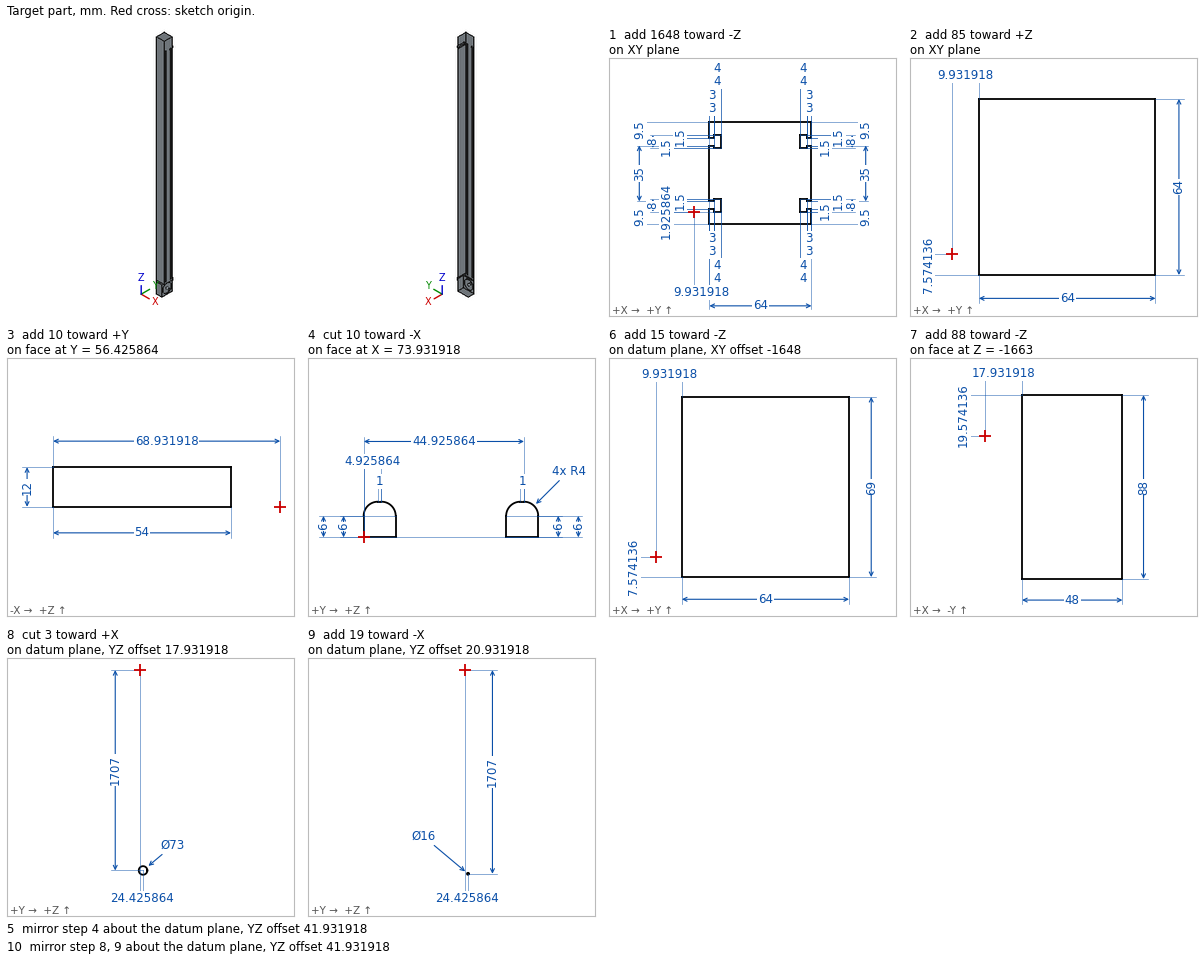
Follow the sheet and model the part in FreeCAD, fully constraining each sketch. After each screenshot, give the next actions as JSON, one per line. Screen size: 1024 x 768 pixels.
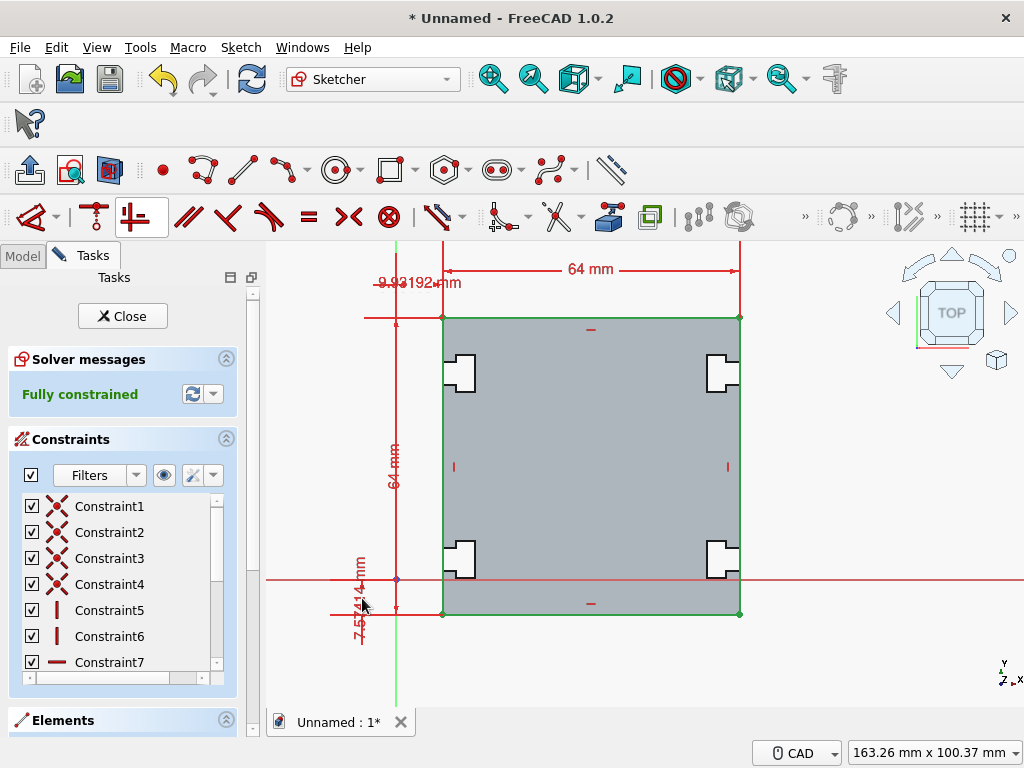
{"action": "left_click", "coordinate": [123, 316]}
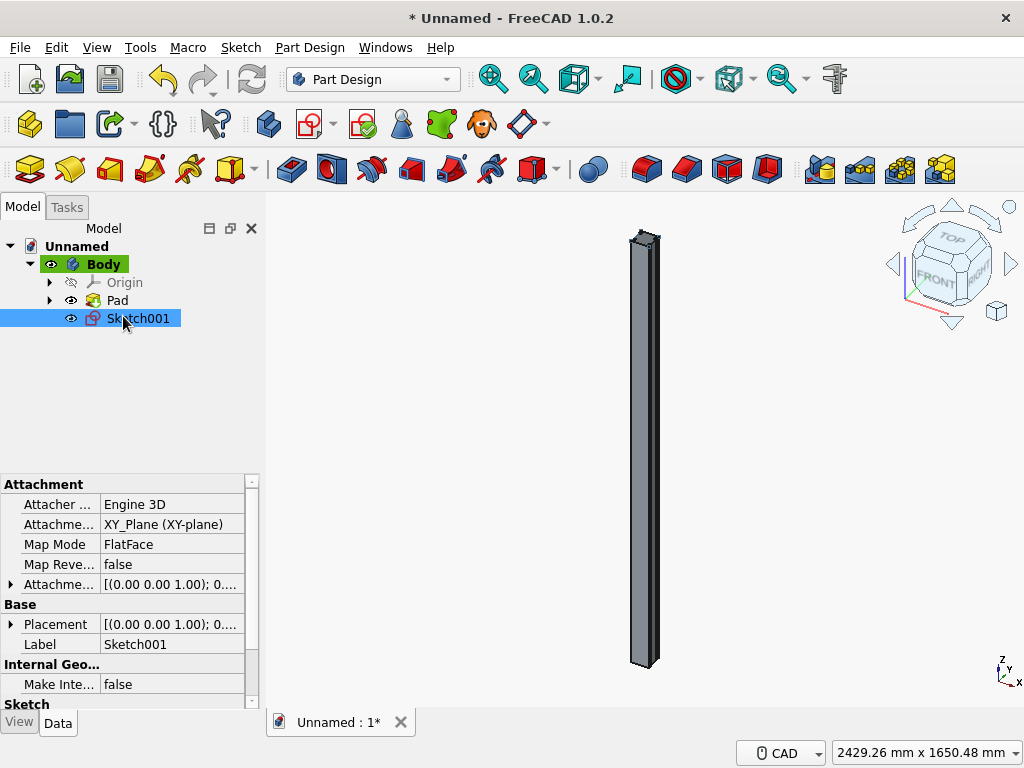
{"action": "left_click", "coordinate": [30, 170]}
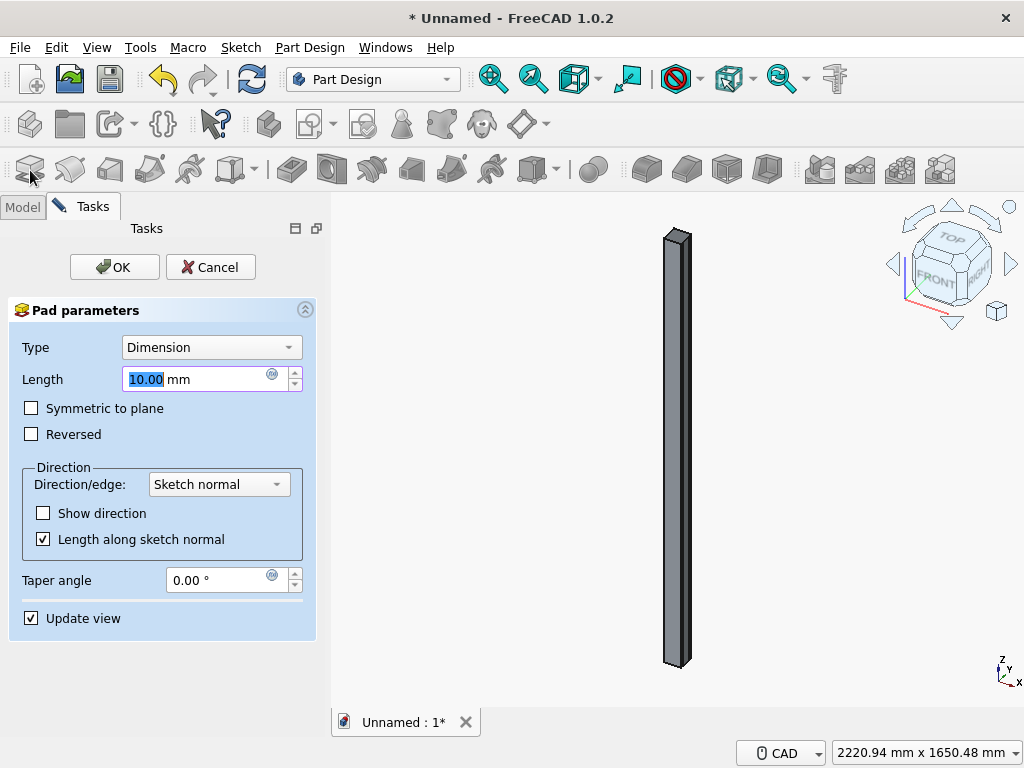
{"action": "type", "text": "85"}
{"action": "key", "text": "Tab"}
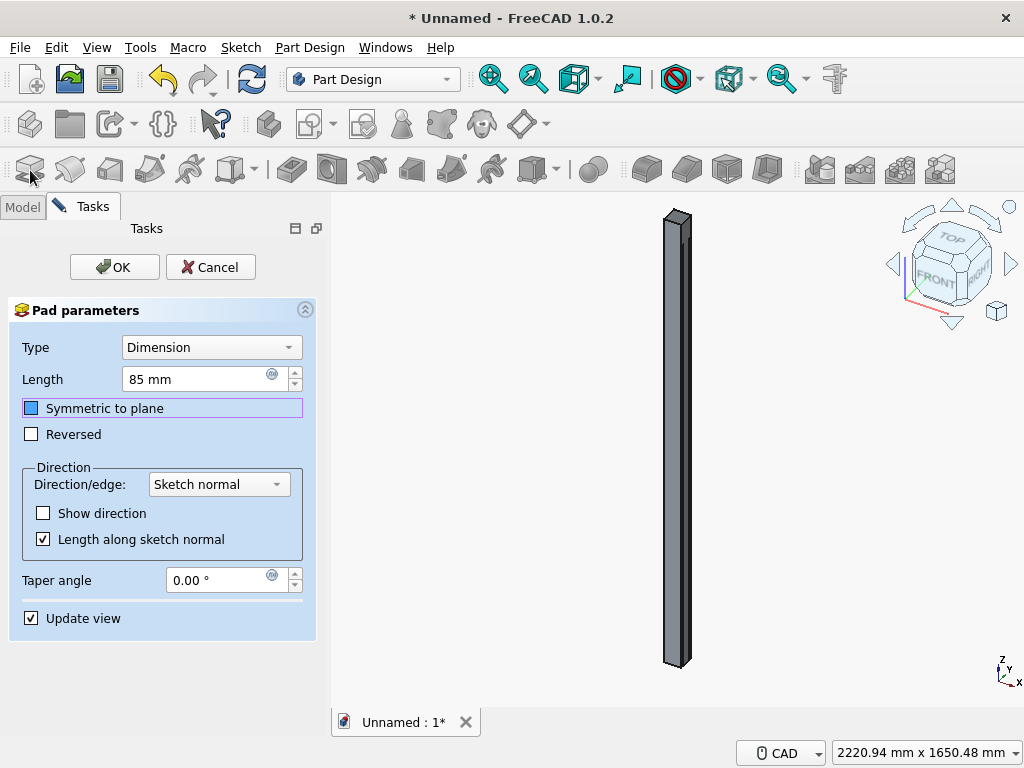
{"action": "left_click", "coordinate": [115, 267]}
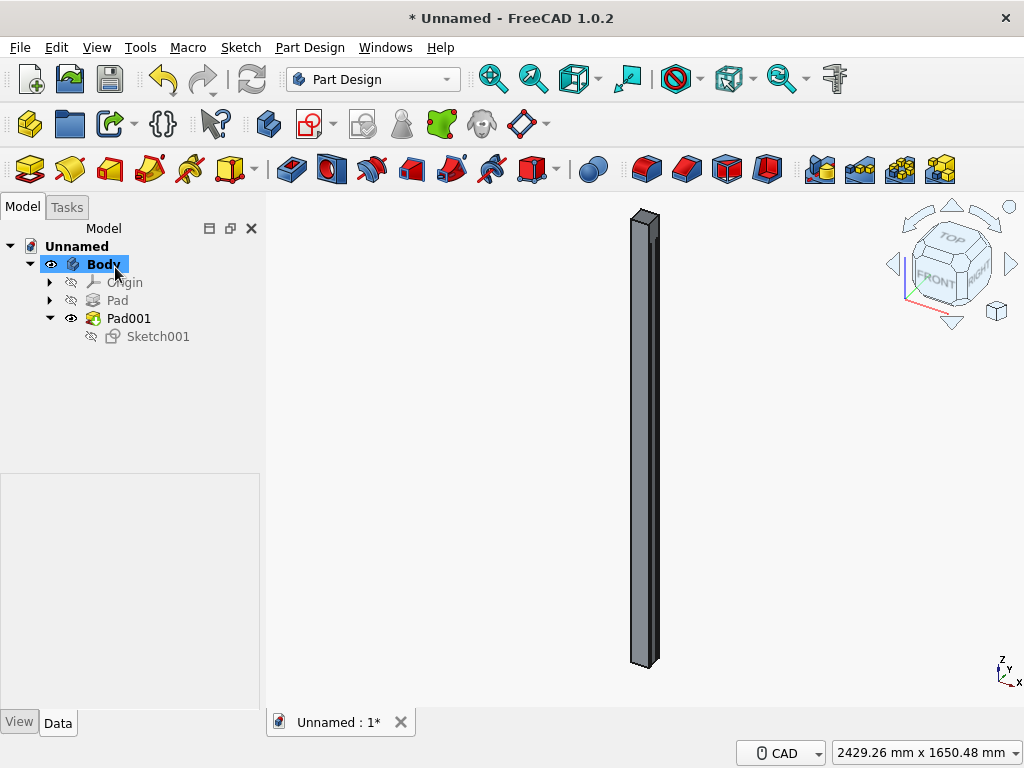
{"action": "key", "text": "4"}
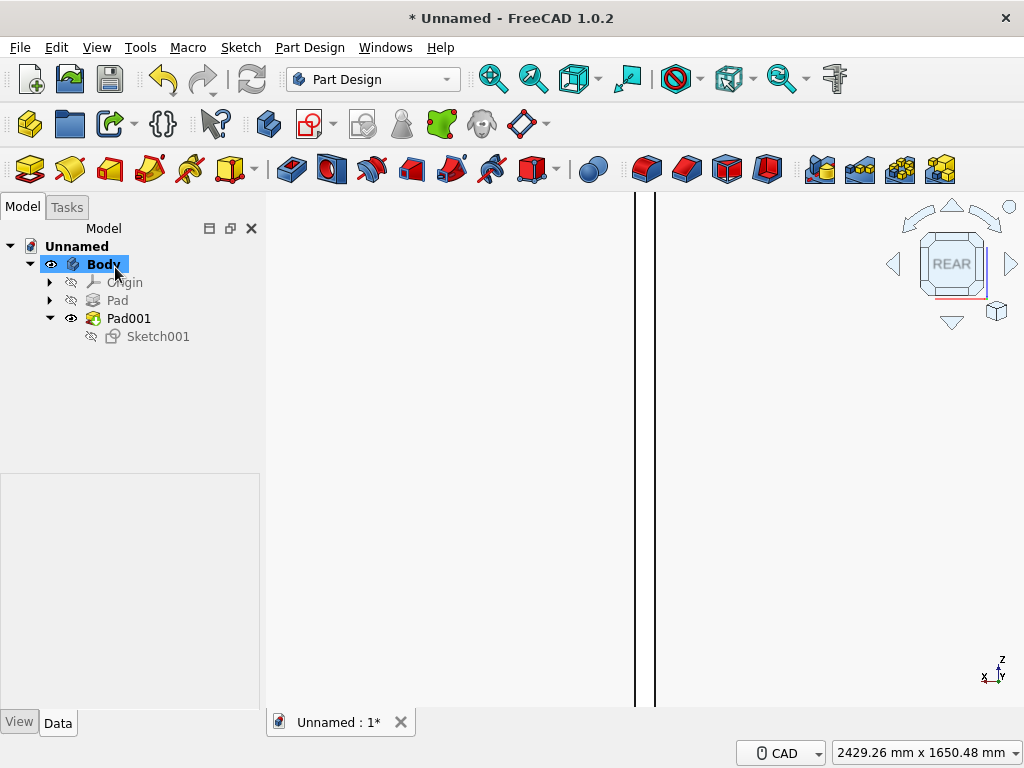
{"action": "left_click", "coordinate": [494, 80]}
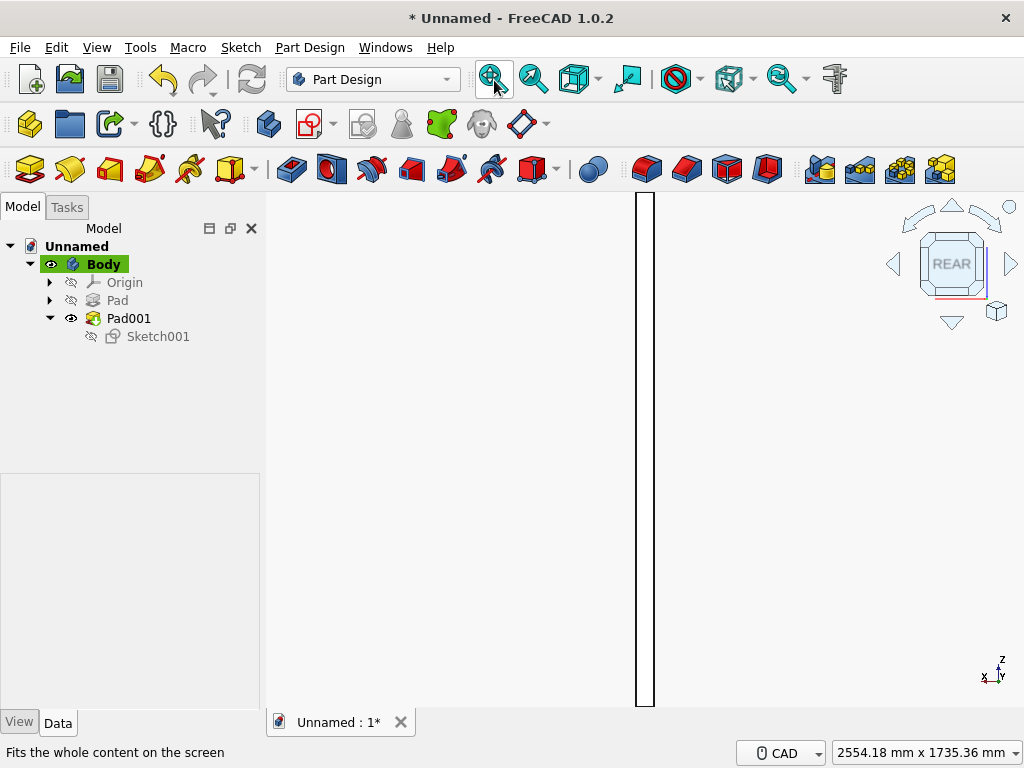
{"action": "left_click", "coordinate": [645, 228]}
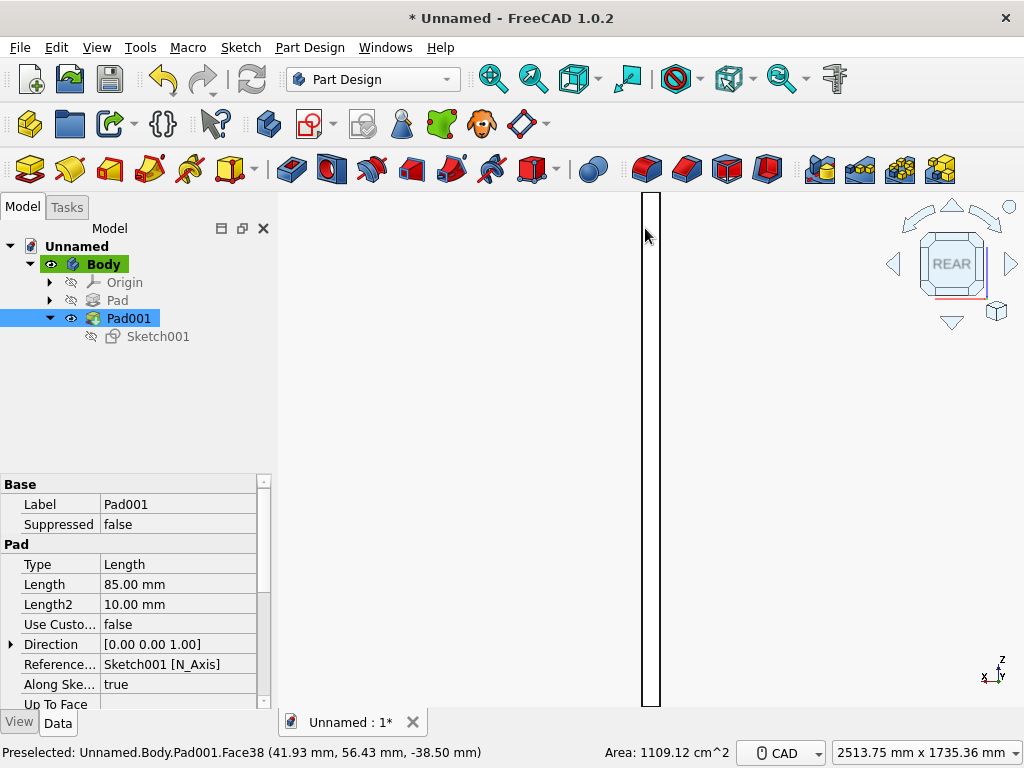
{"action": "left_click", "coordinate": [310, 124]}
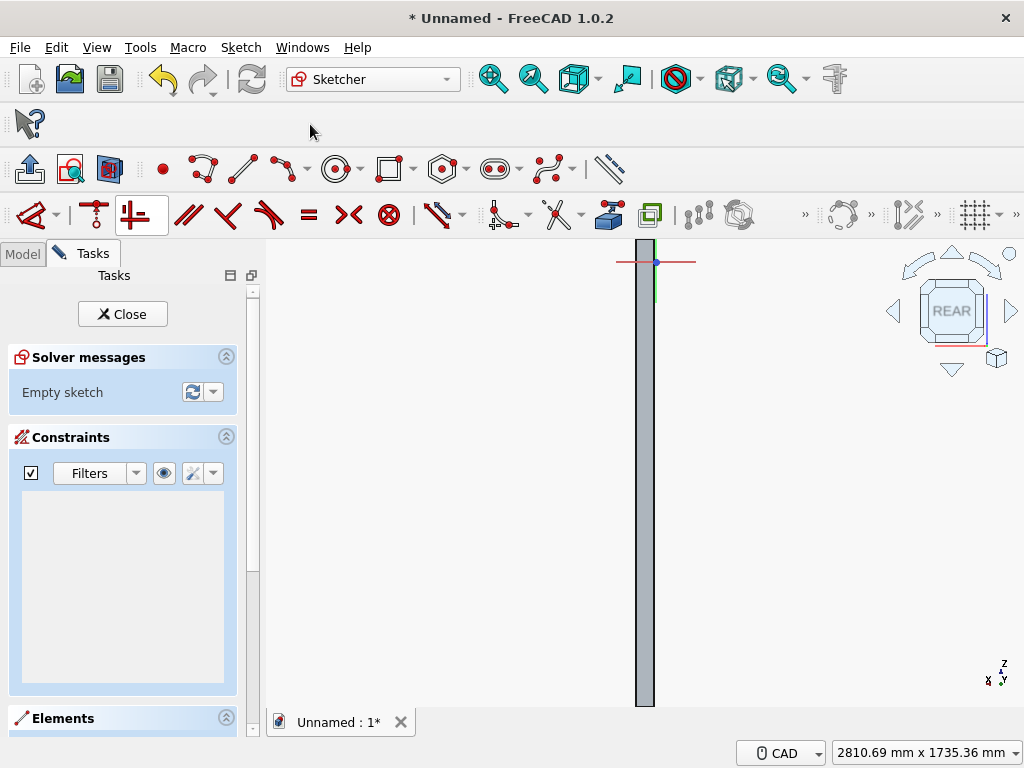
{"action": "scroll", "coordinate": [576, 473], "scroll_direction": "down", "scroll_amount": 5}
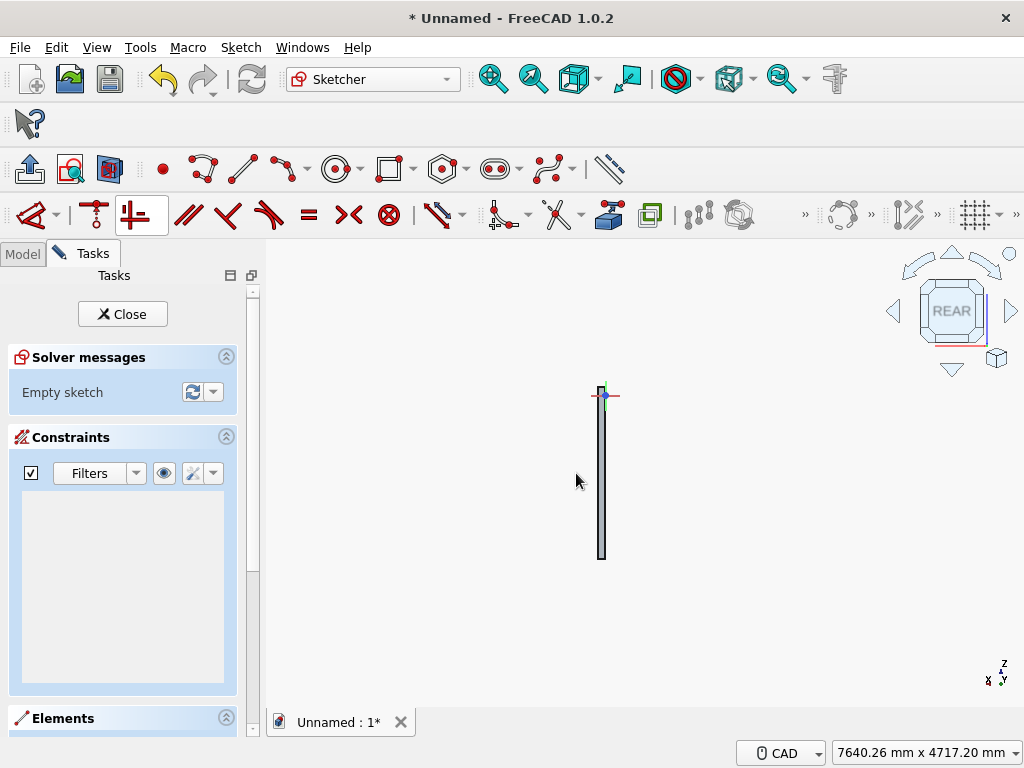
{"action": "scroll", "coordinate": [604, 391], "scroll_direction": "up", "scroll_amount": 15}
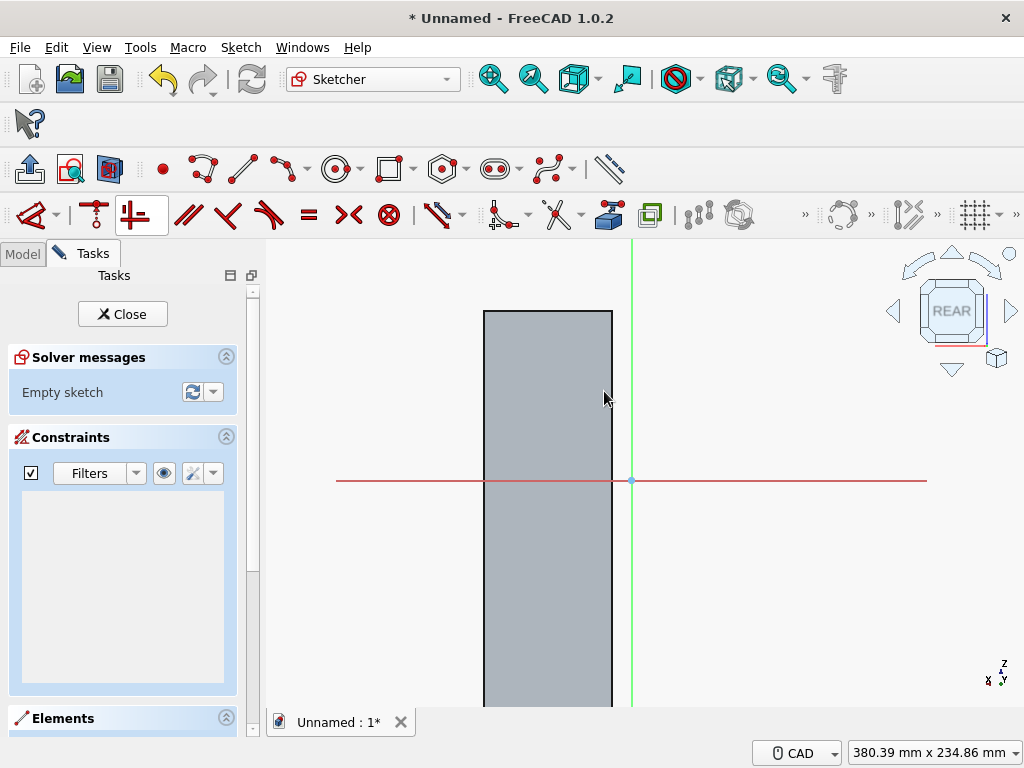
{"action": "scroll", "coordinate": [555, 467], "scroll_direction": "up", "scroll_amount": 5}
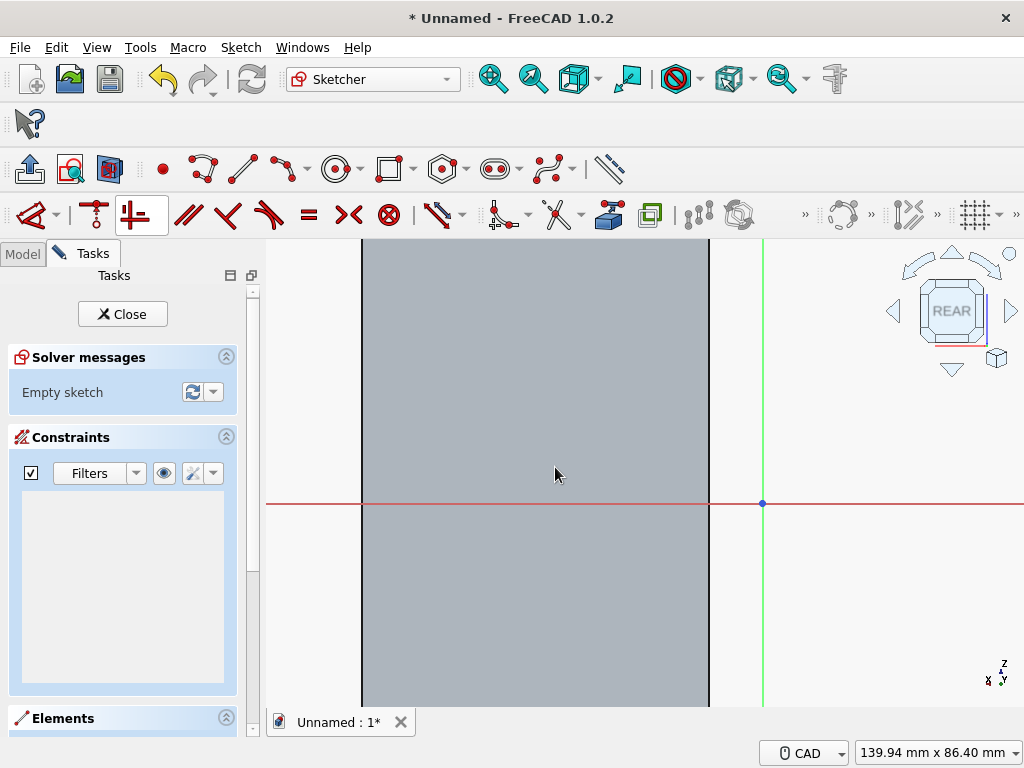
{"action": "left_click", "coordinate": [390, 170]}